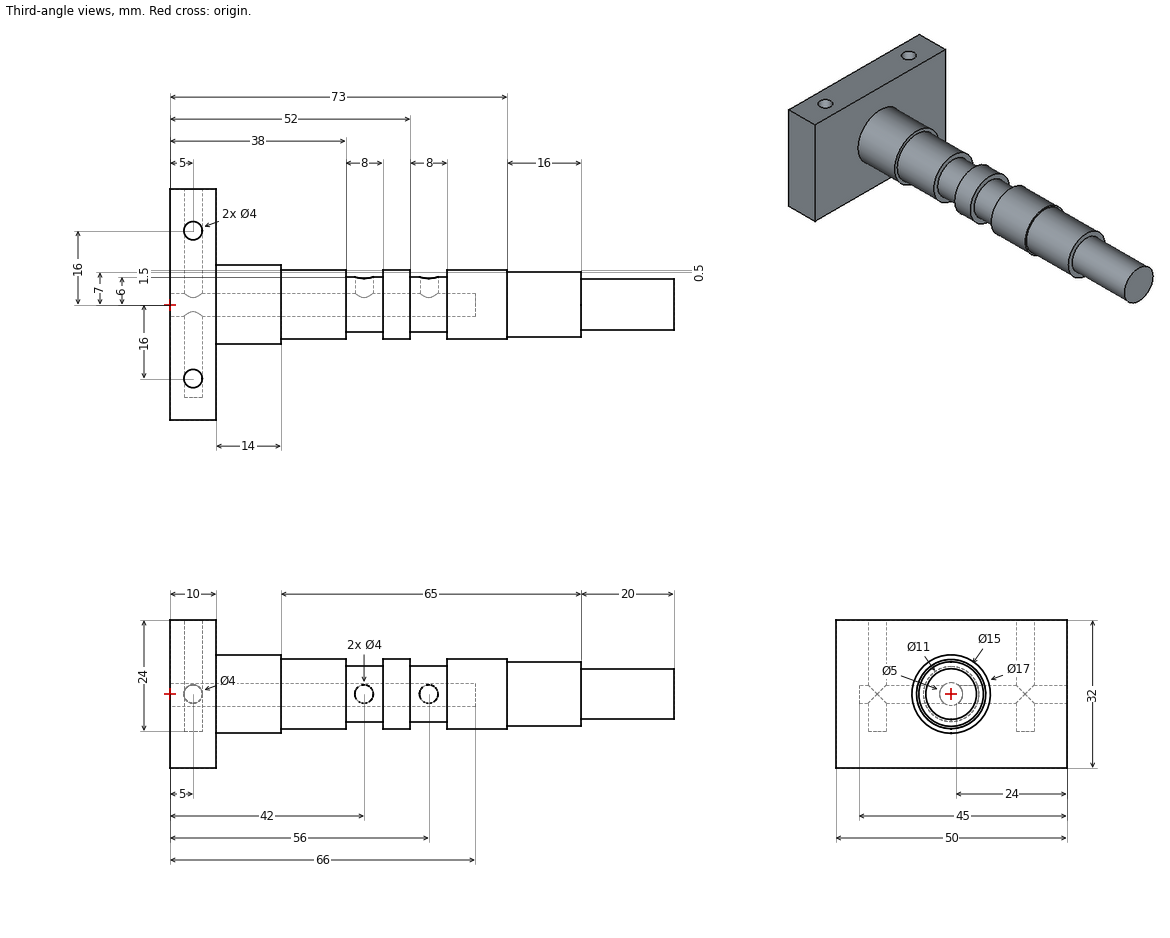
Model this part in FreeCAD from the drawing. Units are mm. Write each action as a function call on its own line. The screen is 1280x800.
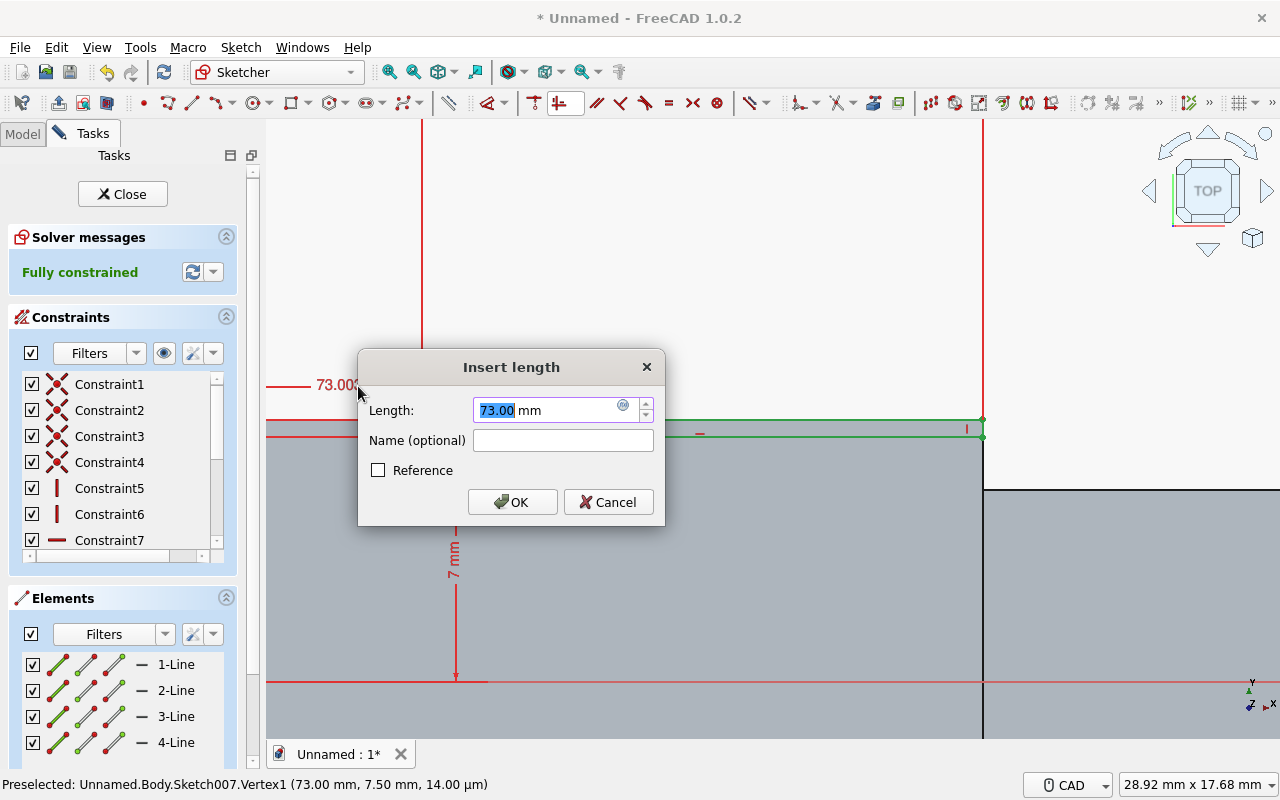
text(73)
key(Return)
key(Escape)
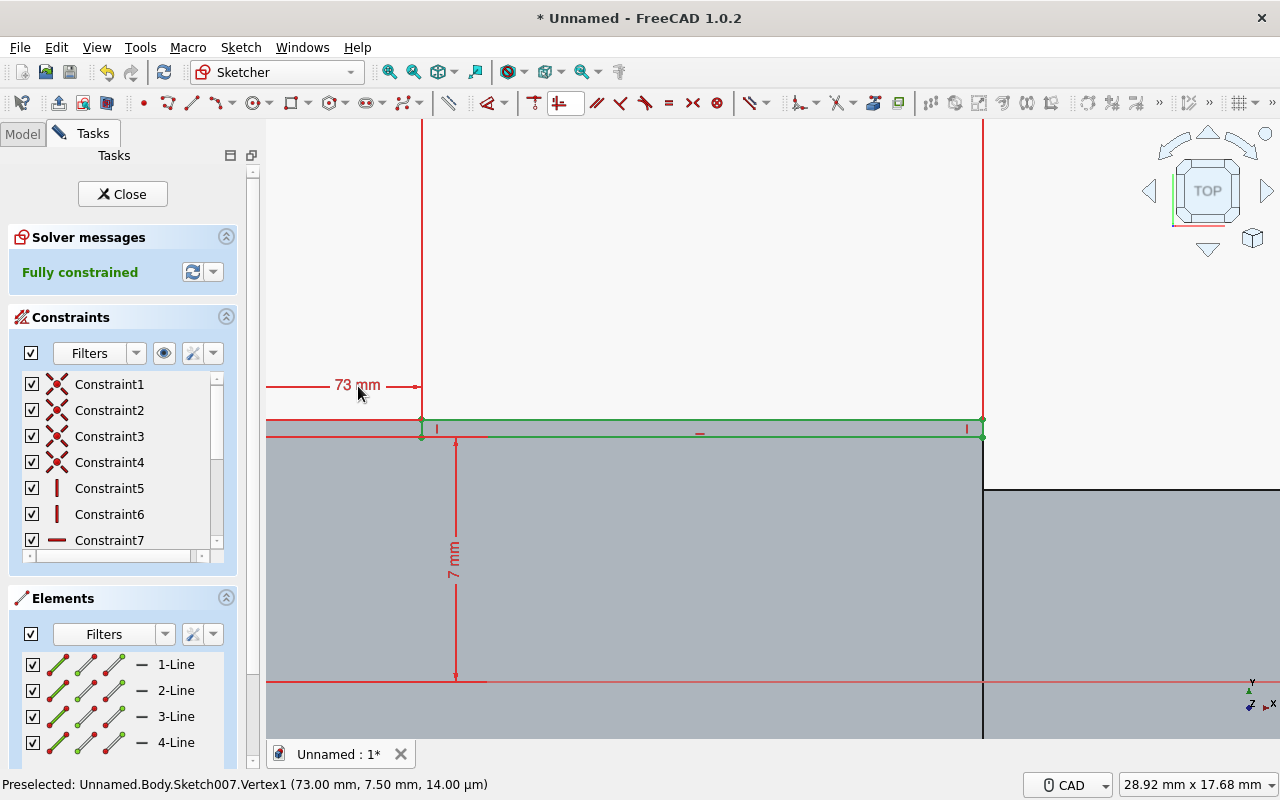
click(123, 194)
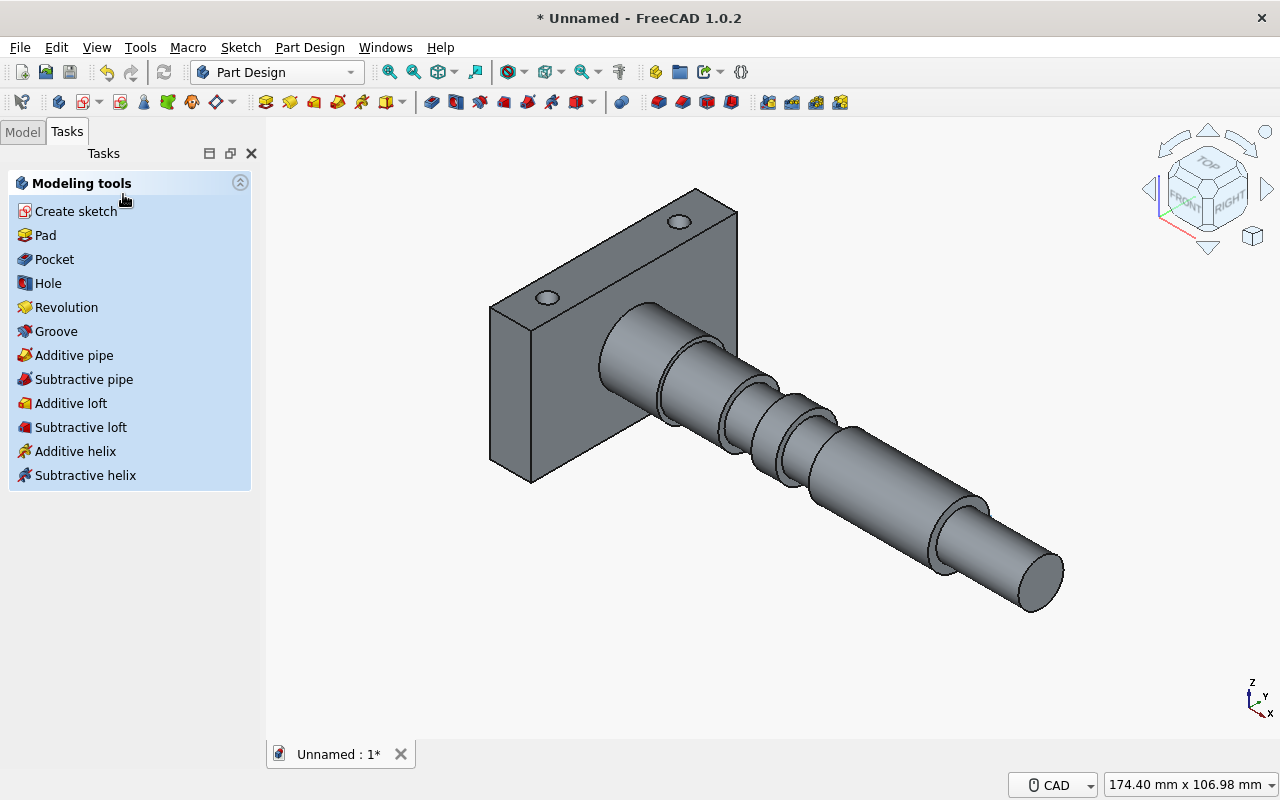
click(480, 102)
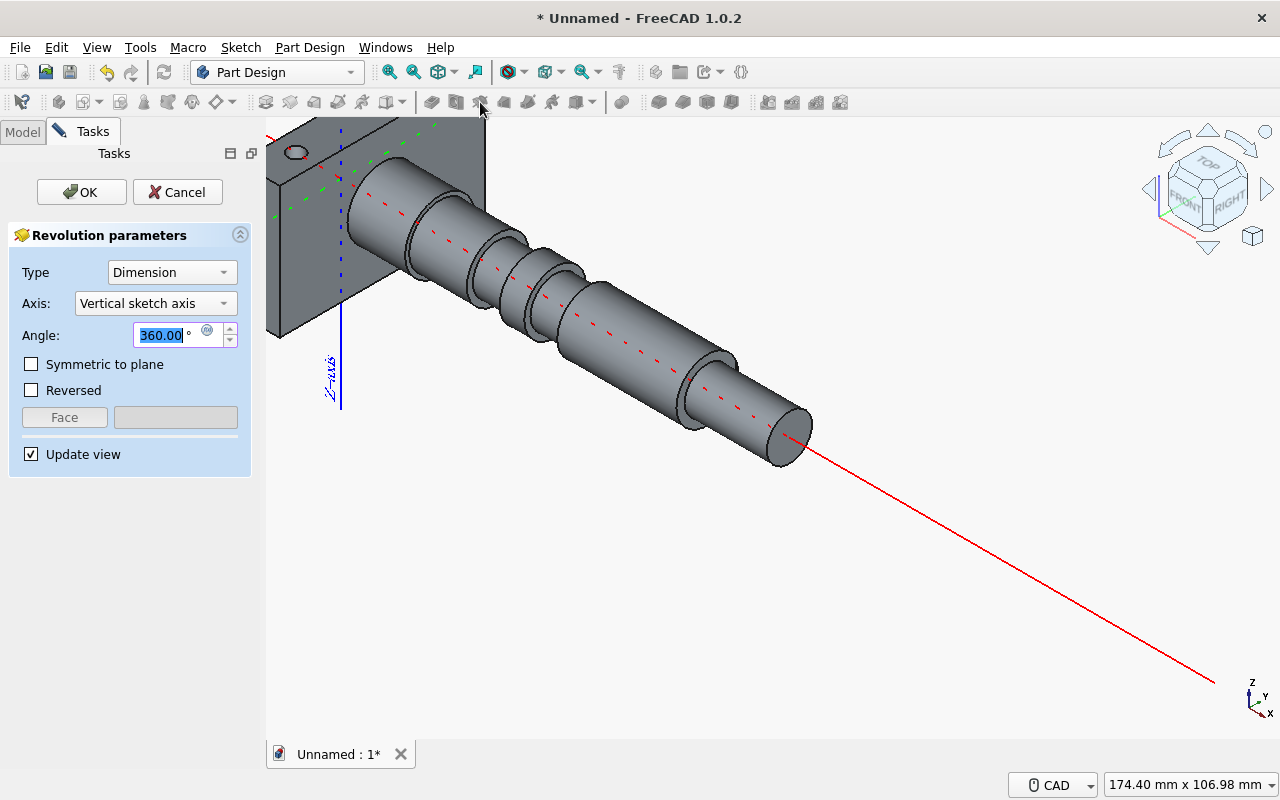
click(156, 304)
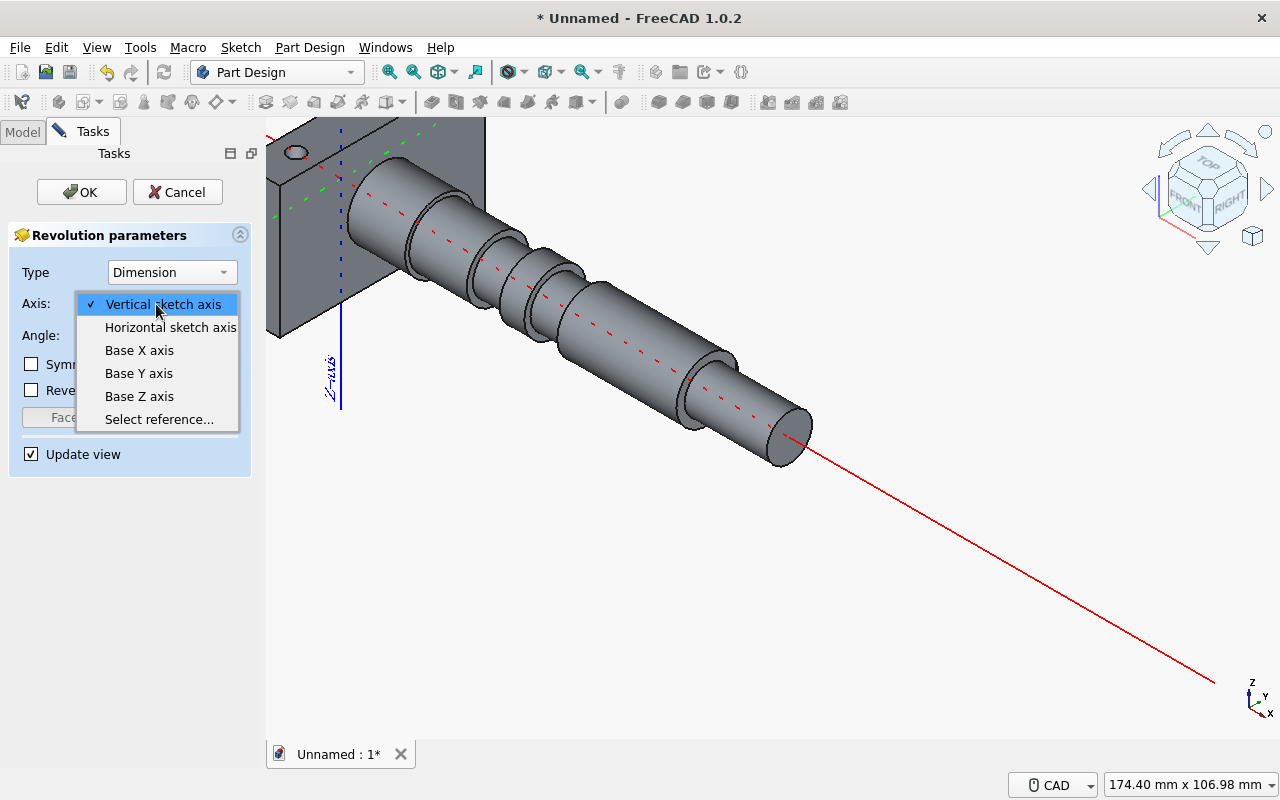
click(156, 328)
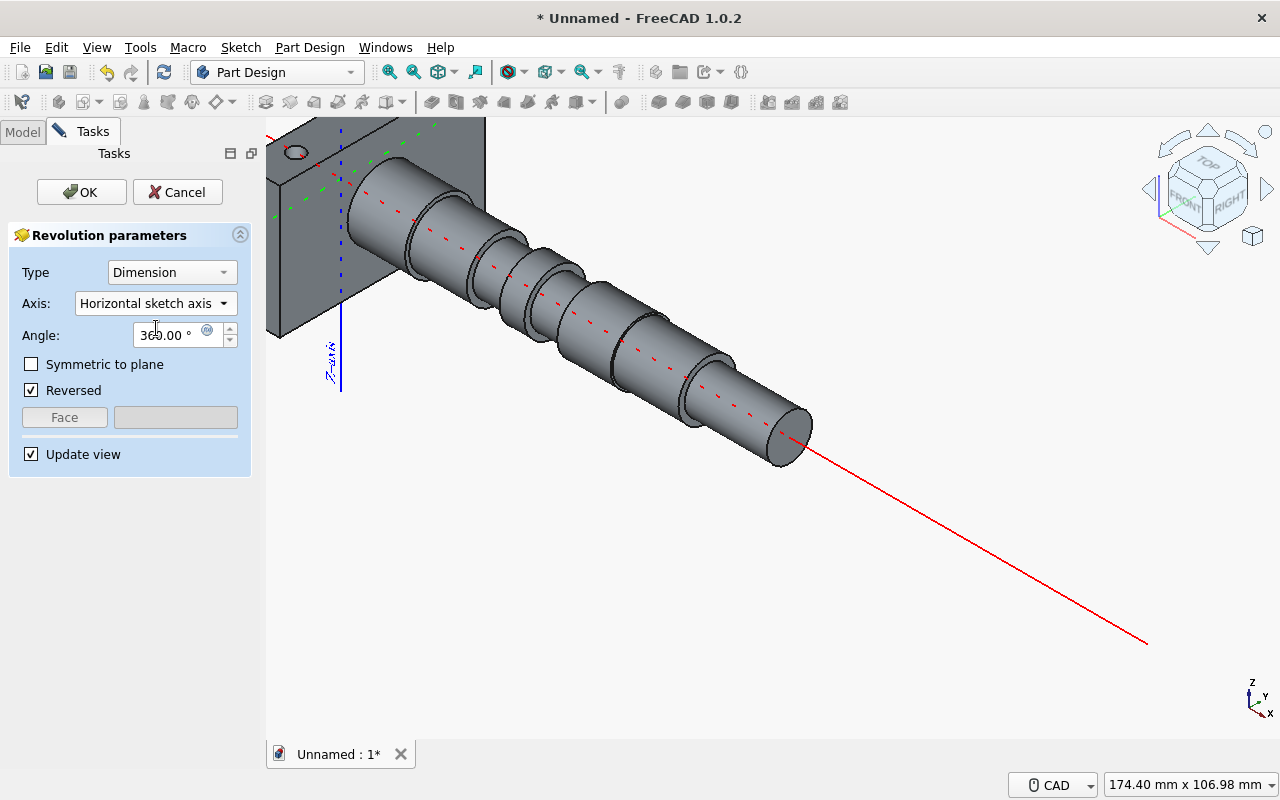
click(82, 192)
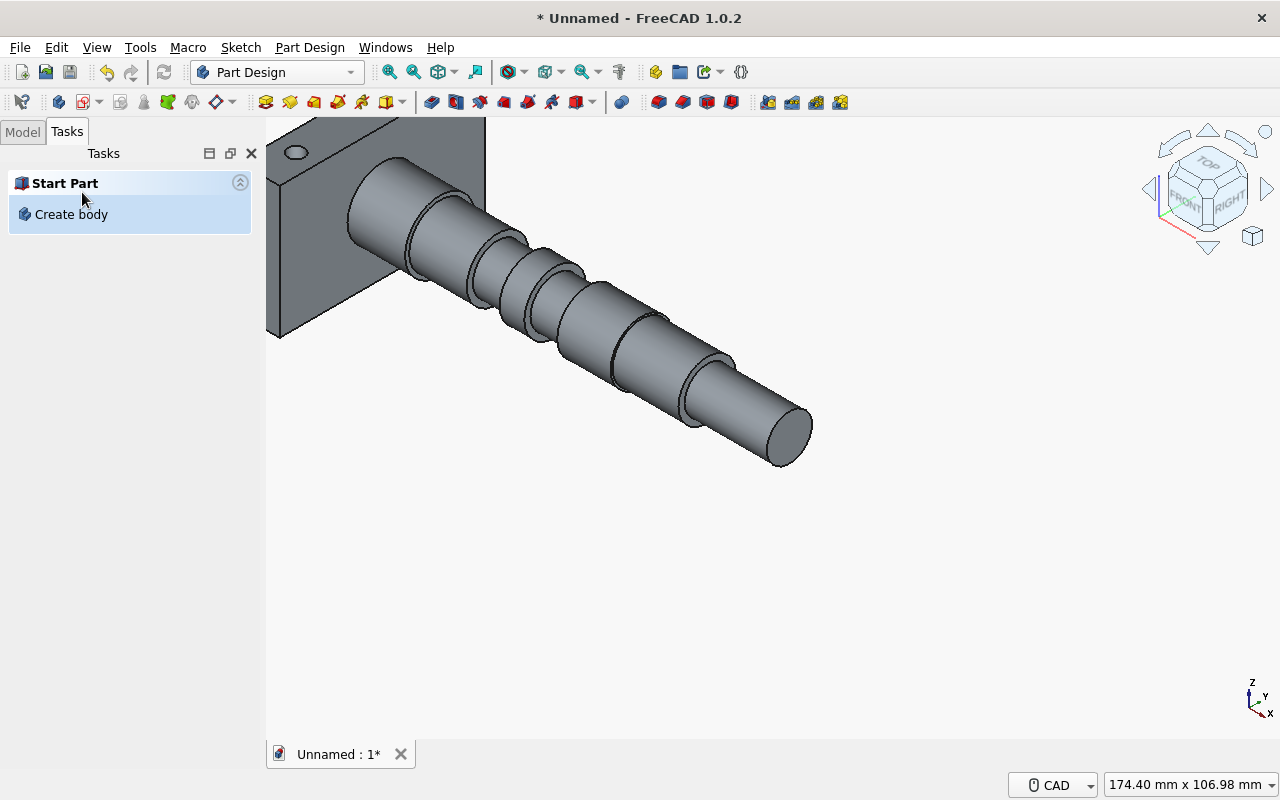
click(390, 72)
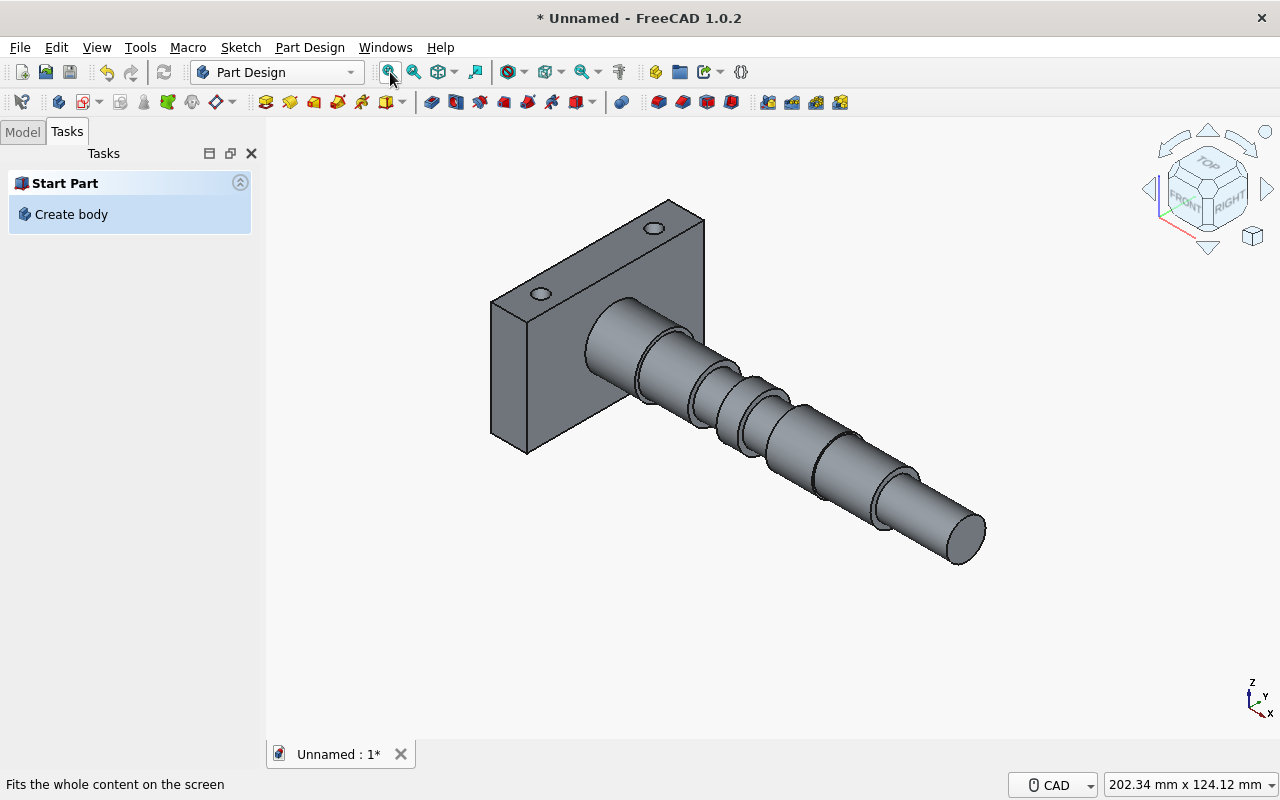
key(6)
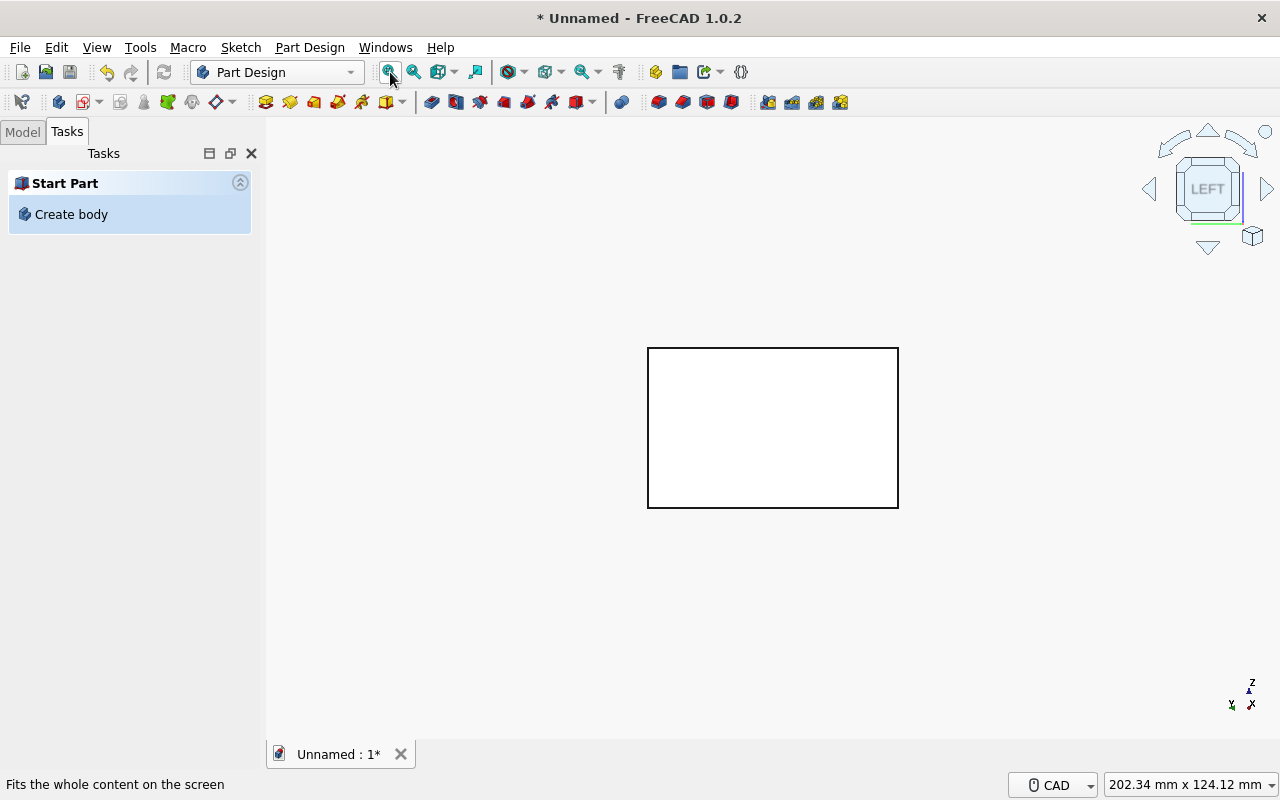
click(390, 72)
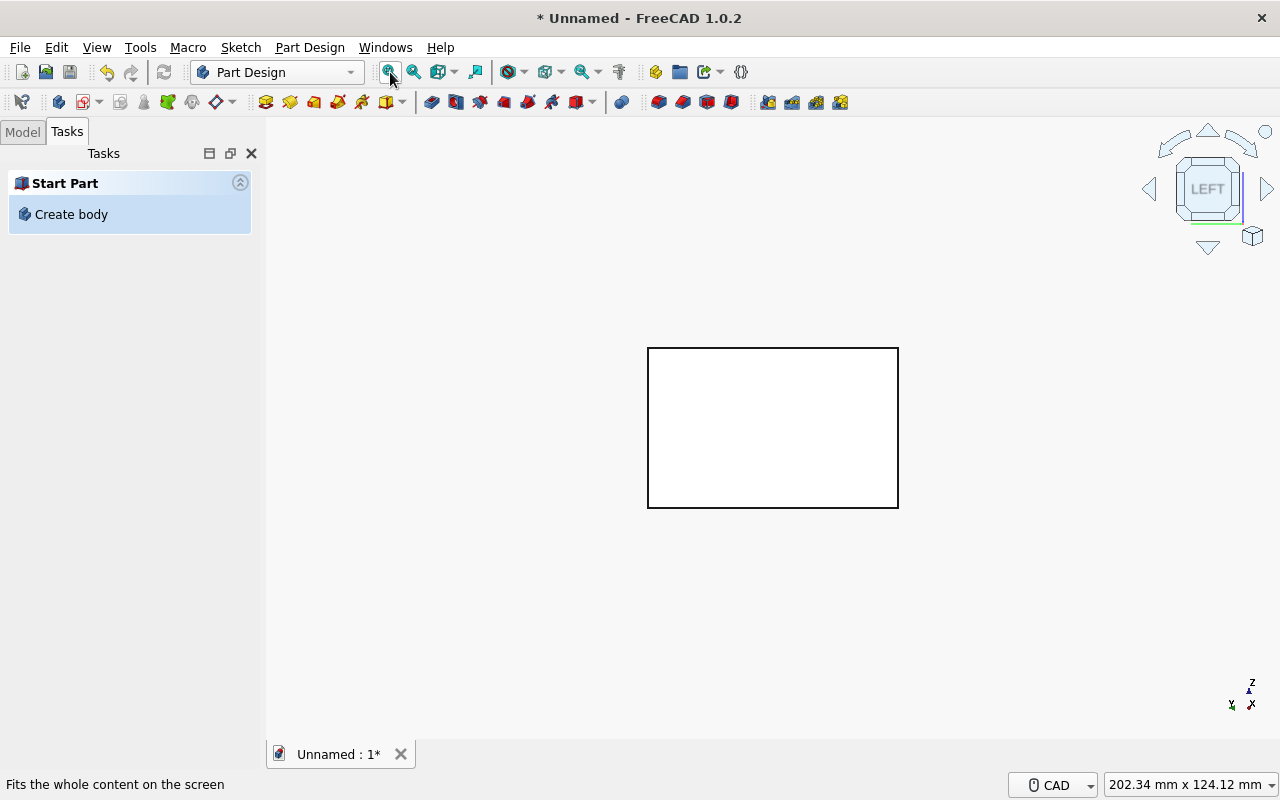
click(773, 427)